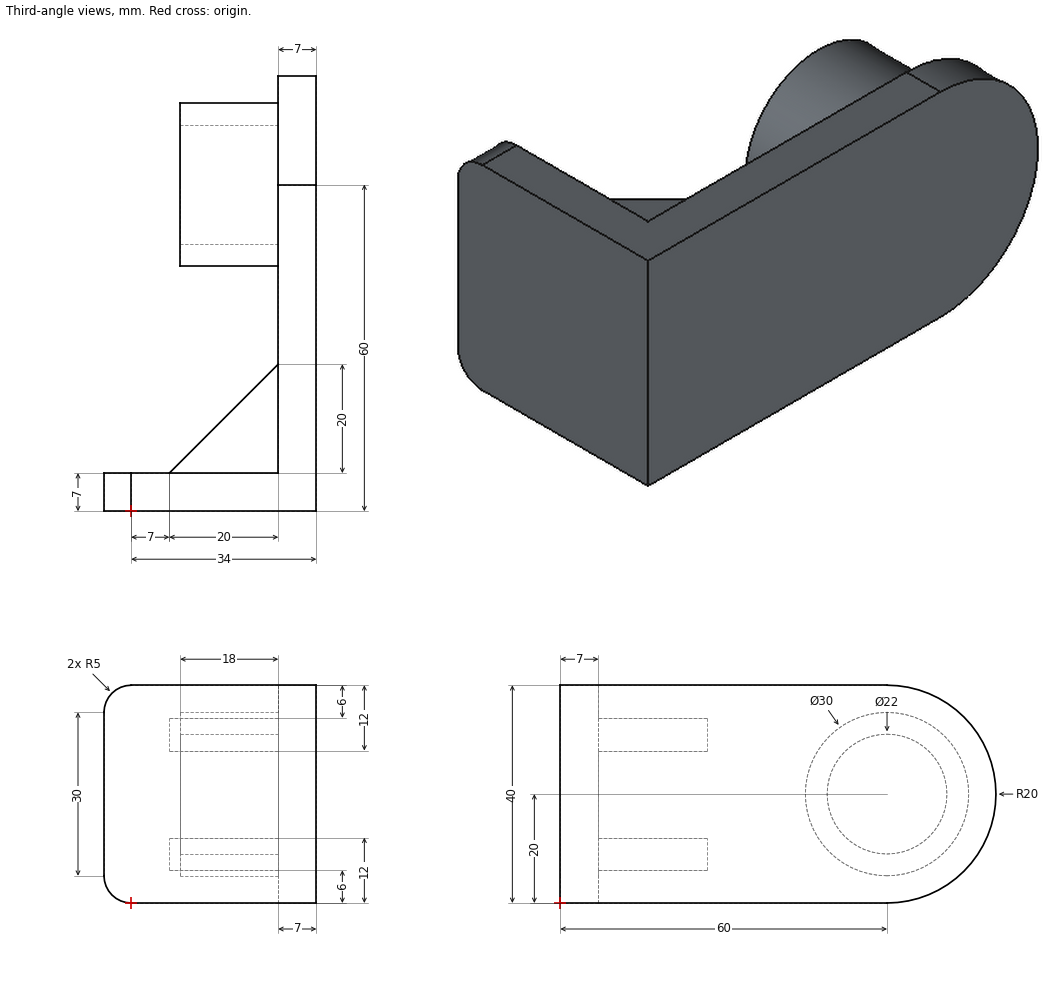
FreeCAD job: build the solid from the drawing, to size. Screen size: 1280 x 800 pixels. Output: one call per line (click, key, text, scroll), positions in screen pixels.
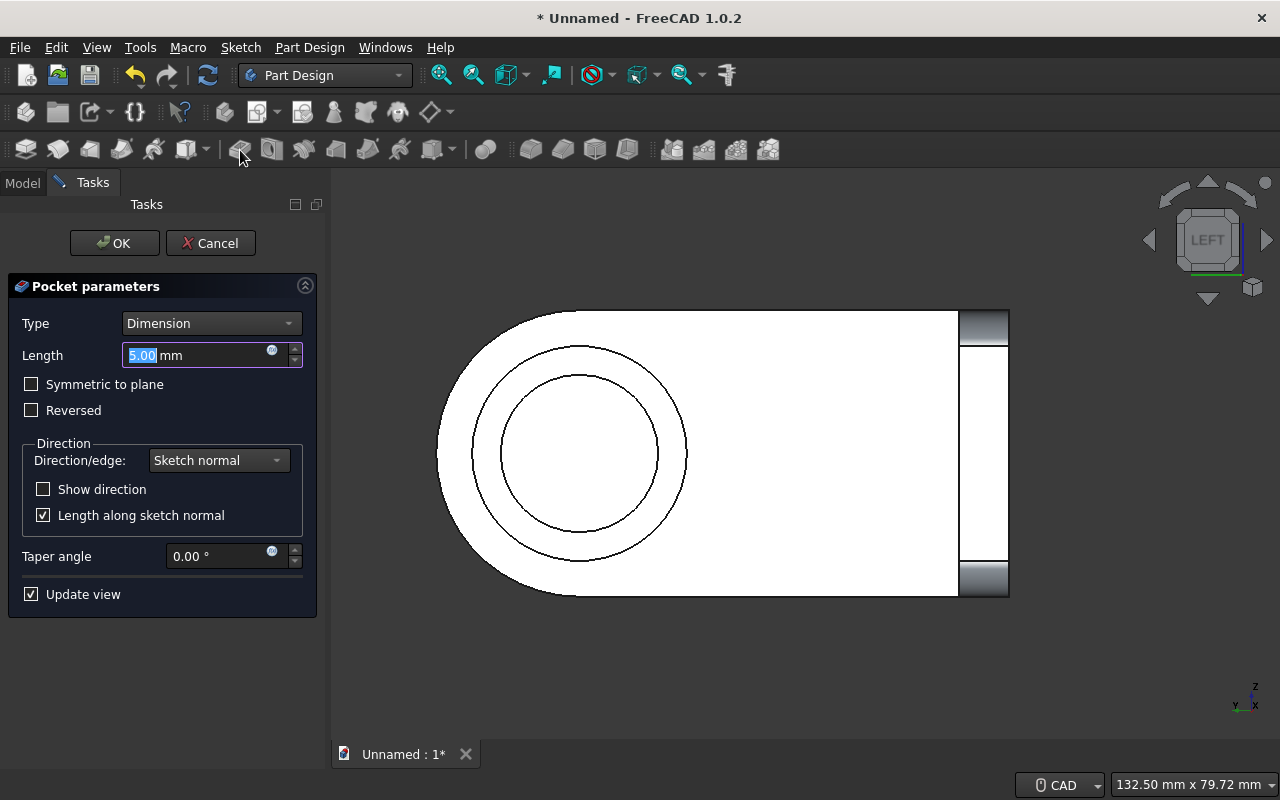
text(18)
key(Tab)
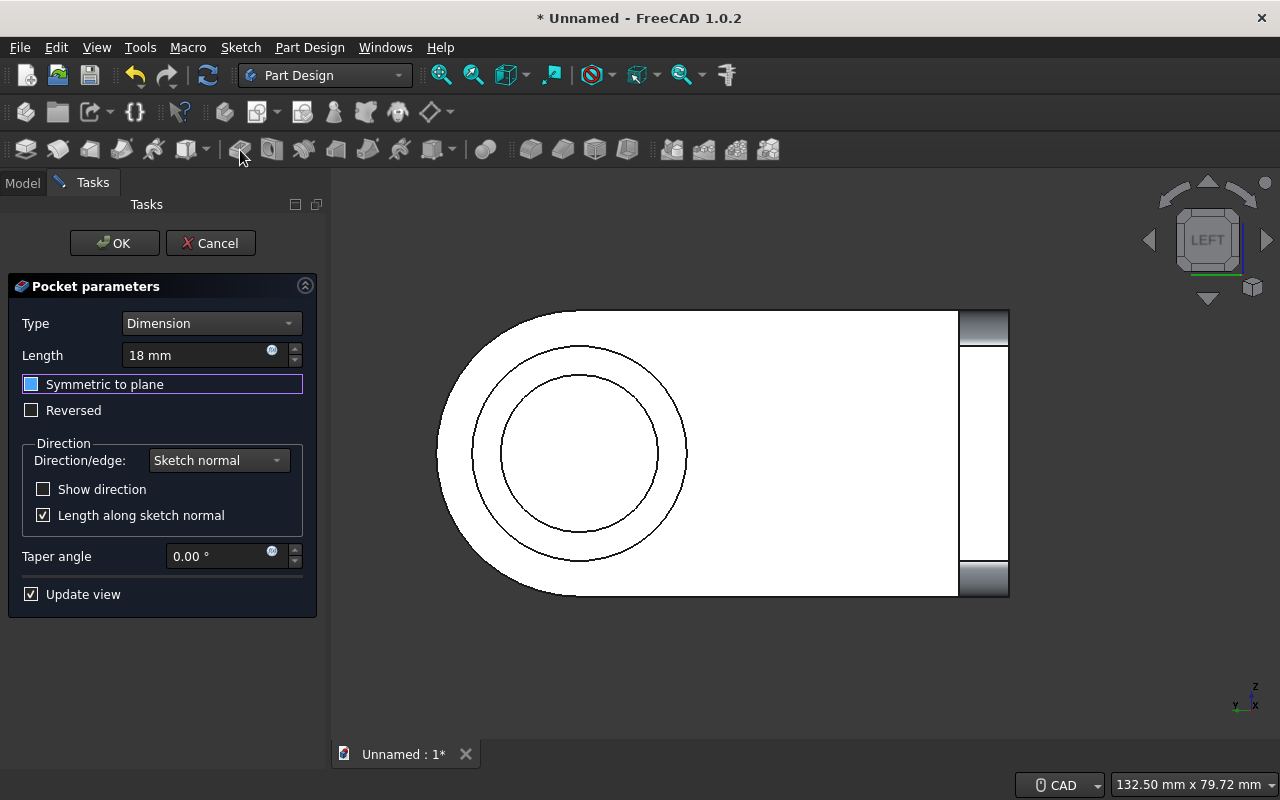
click(115, 243)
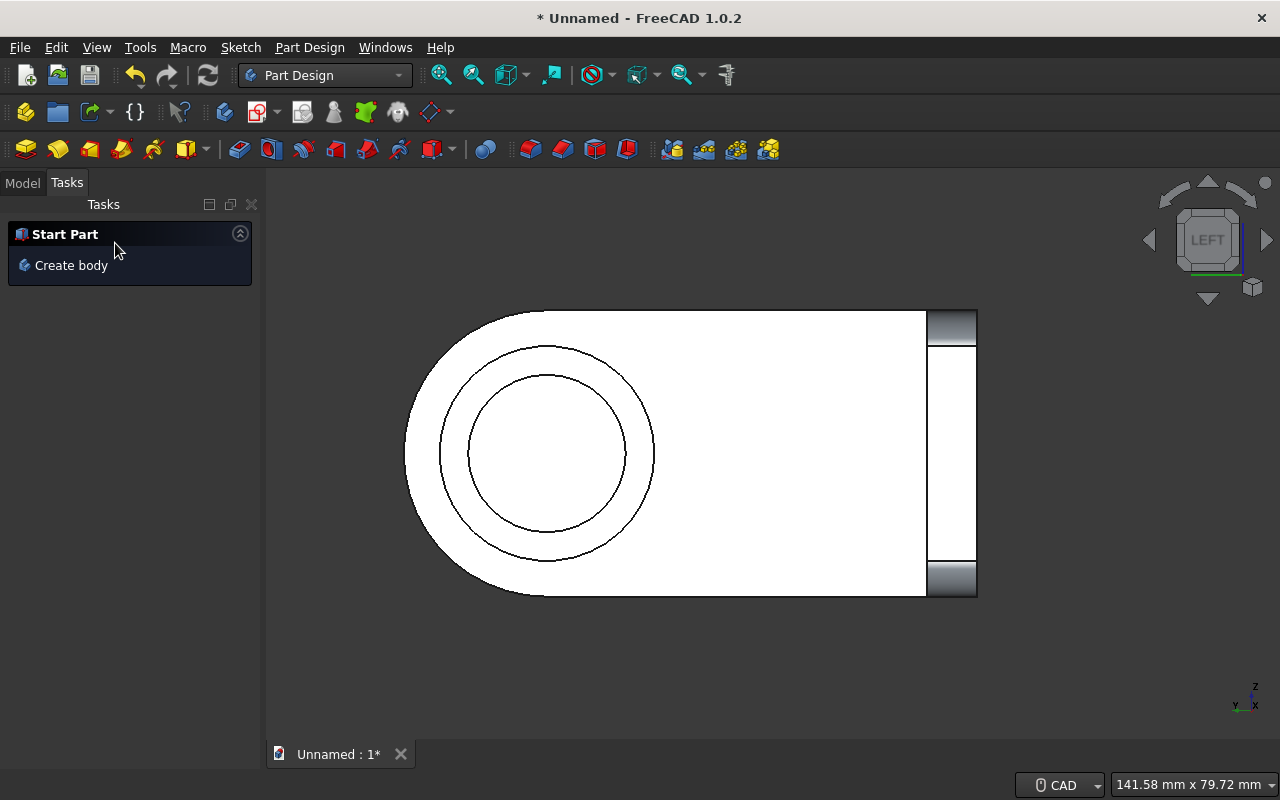
key(0)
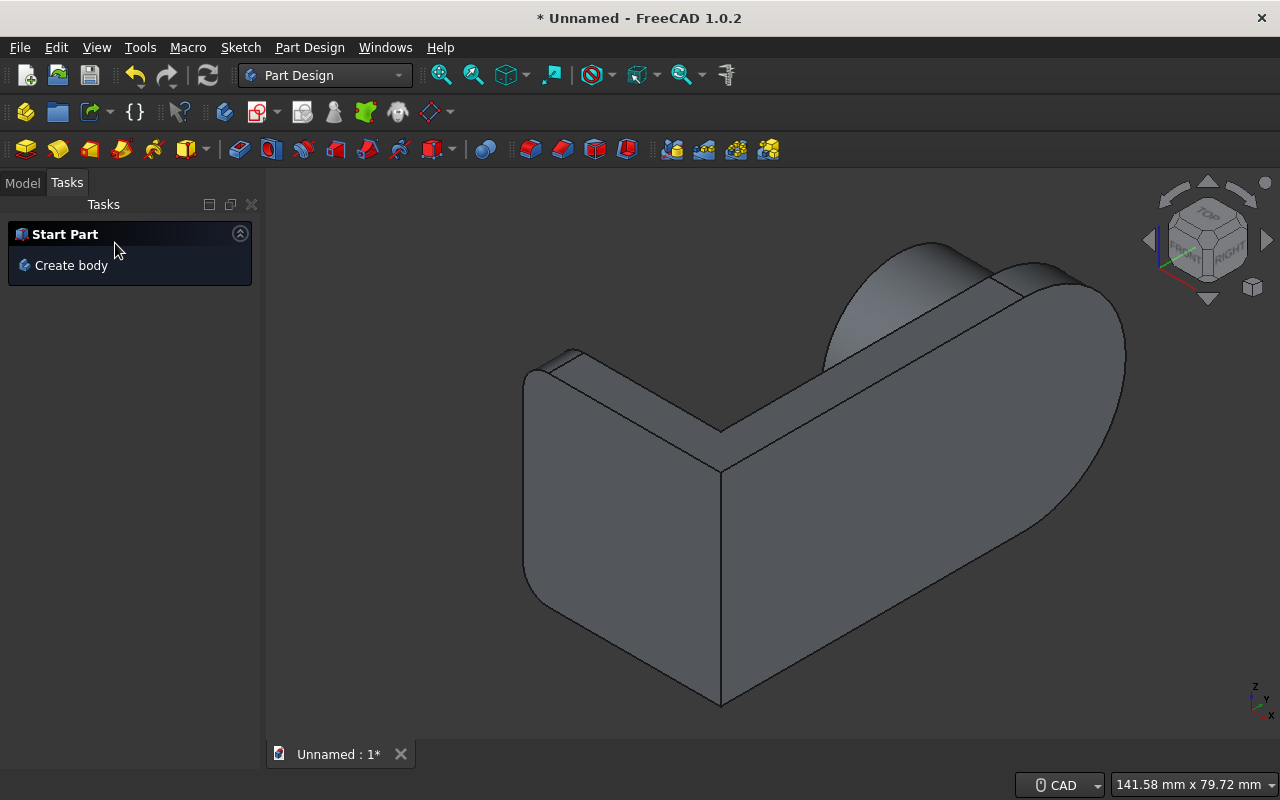
click(442, 76)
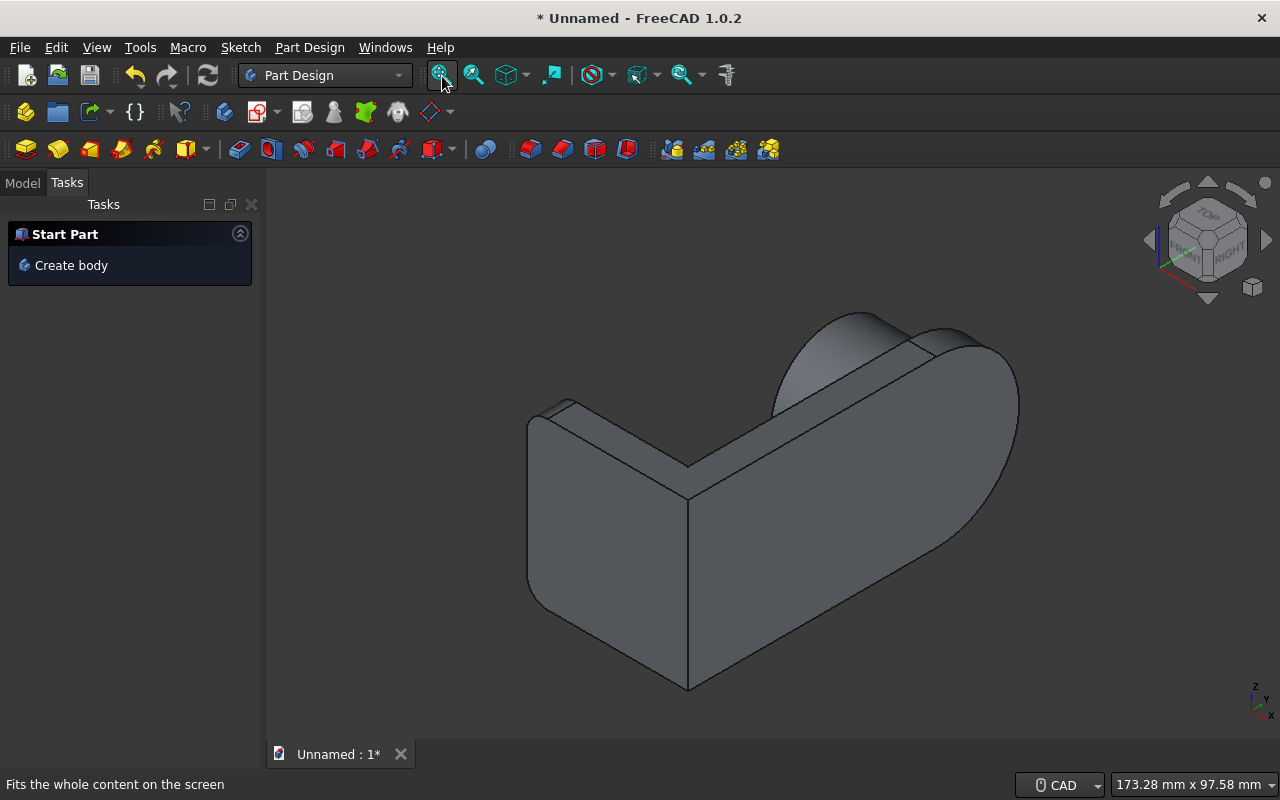
click(676, 471)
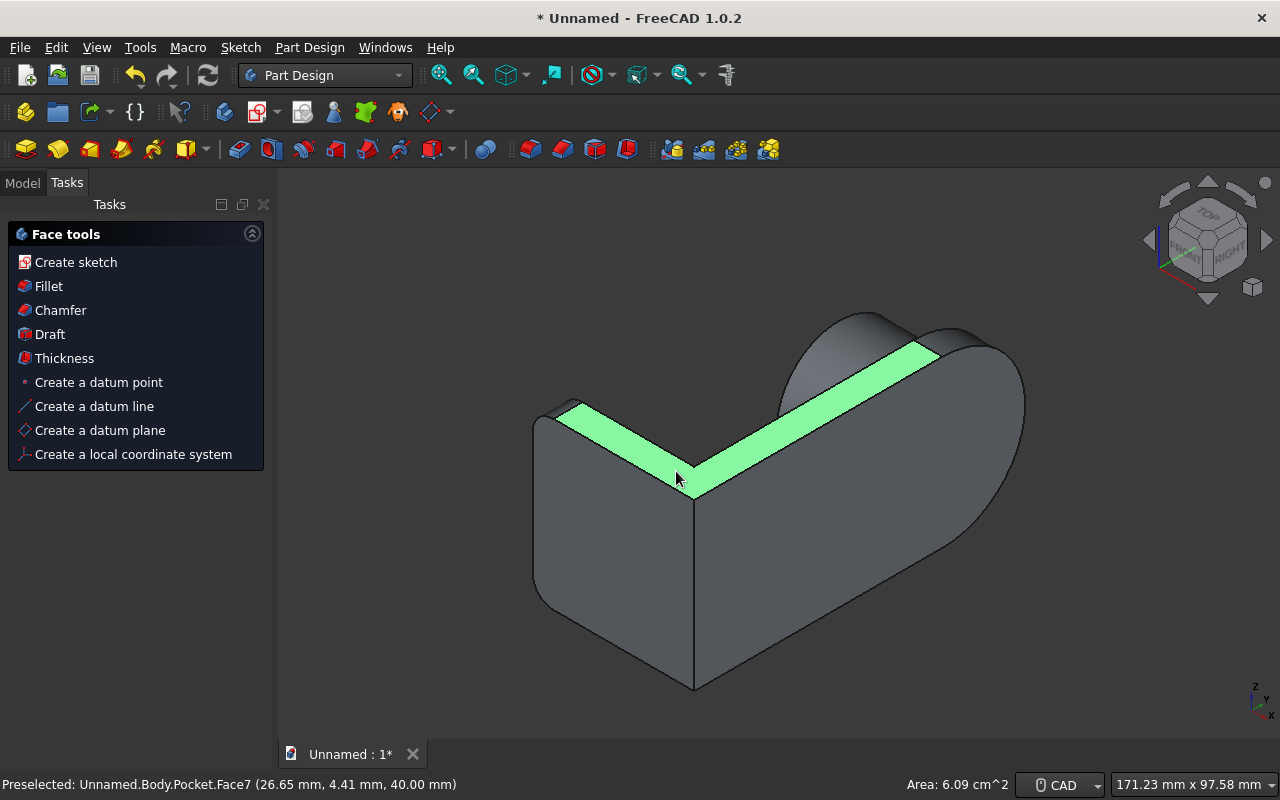
click(258, 112)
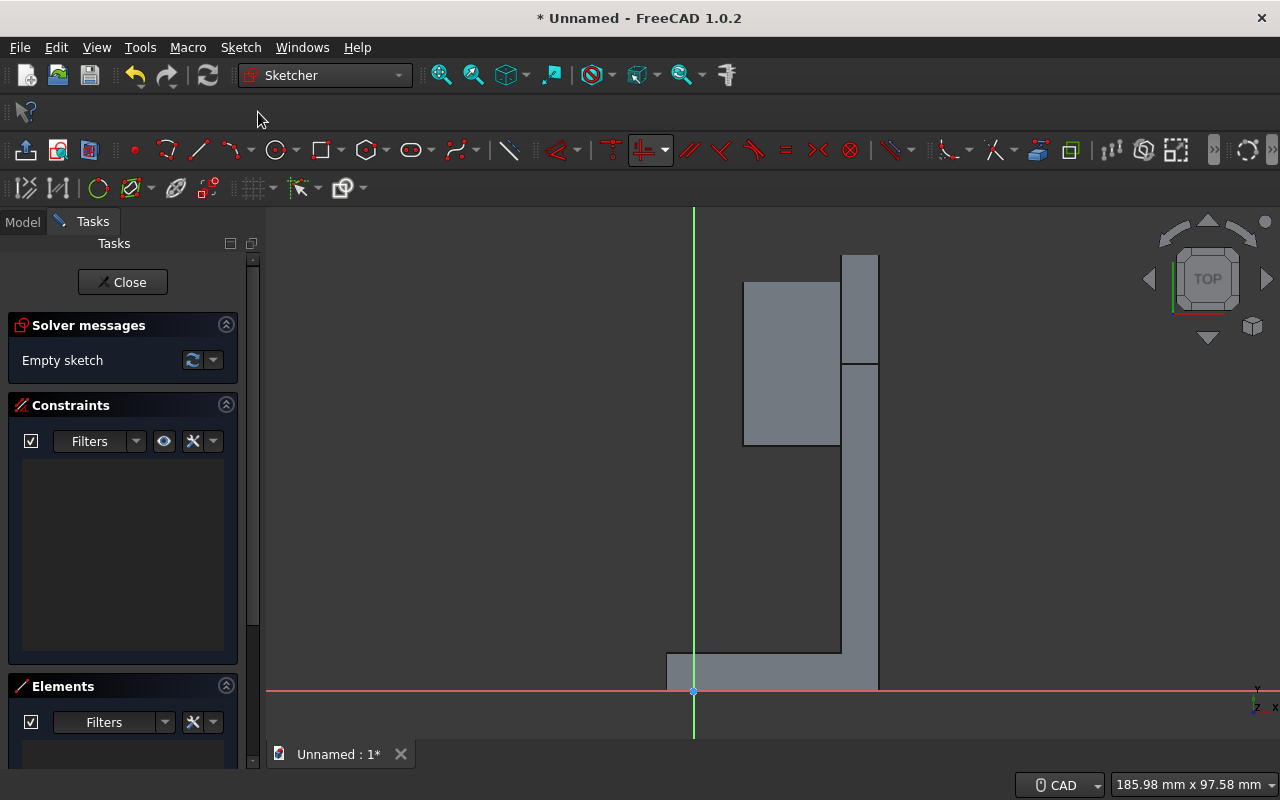
scroll(819, 711, up, 4)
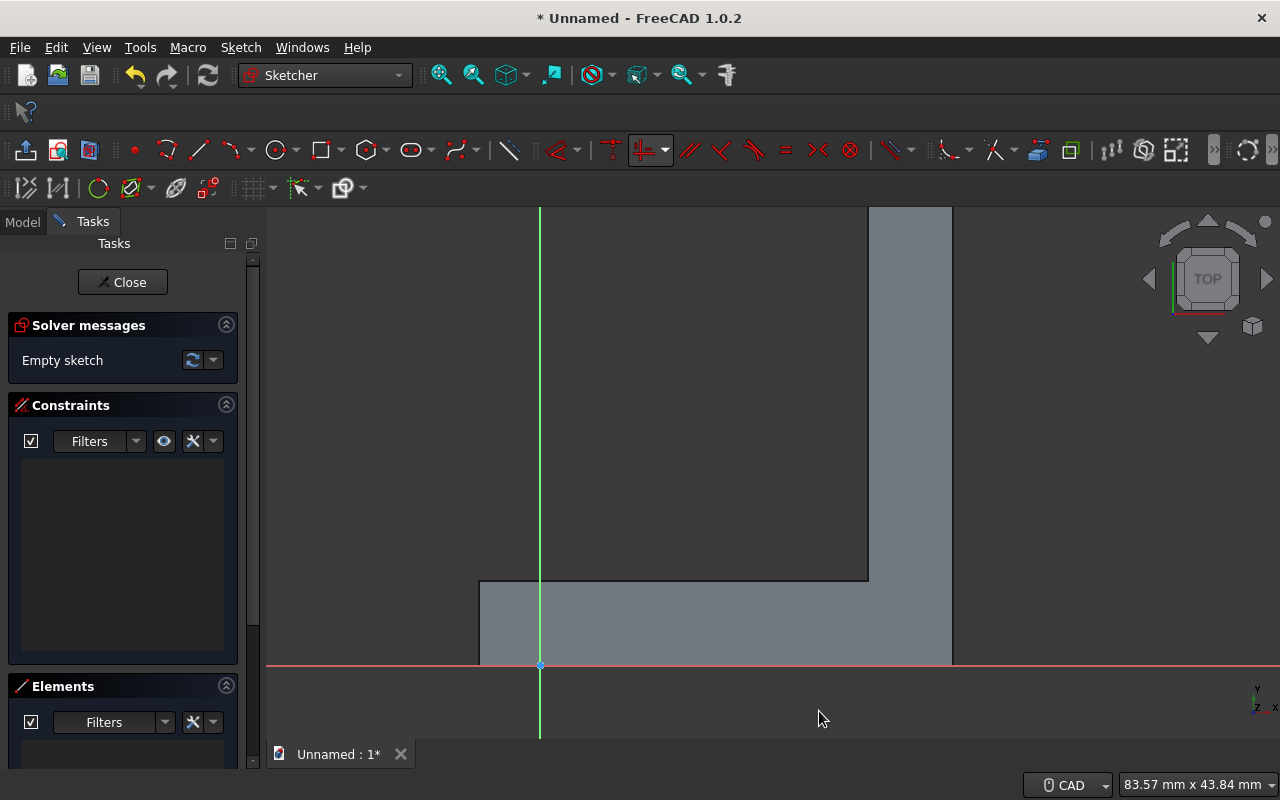
click(168, 150)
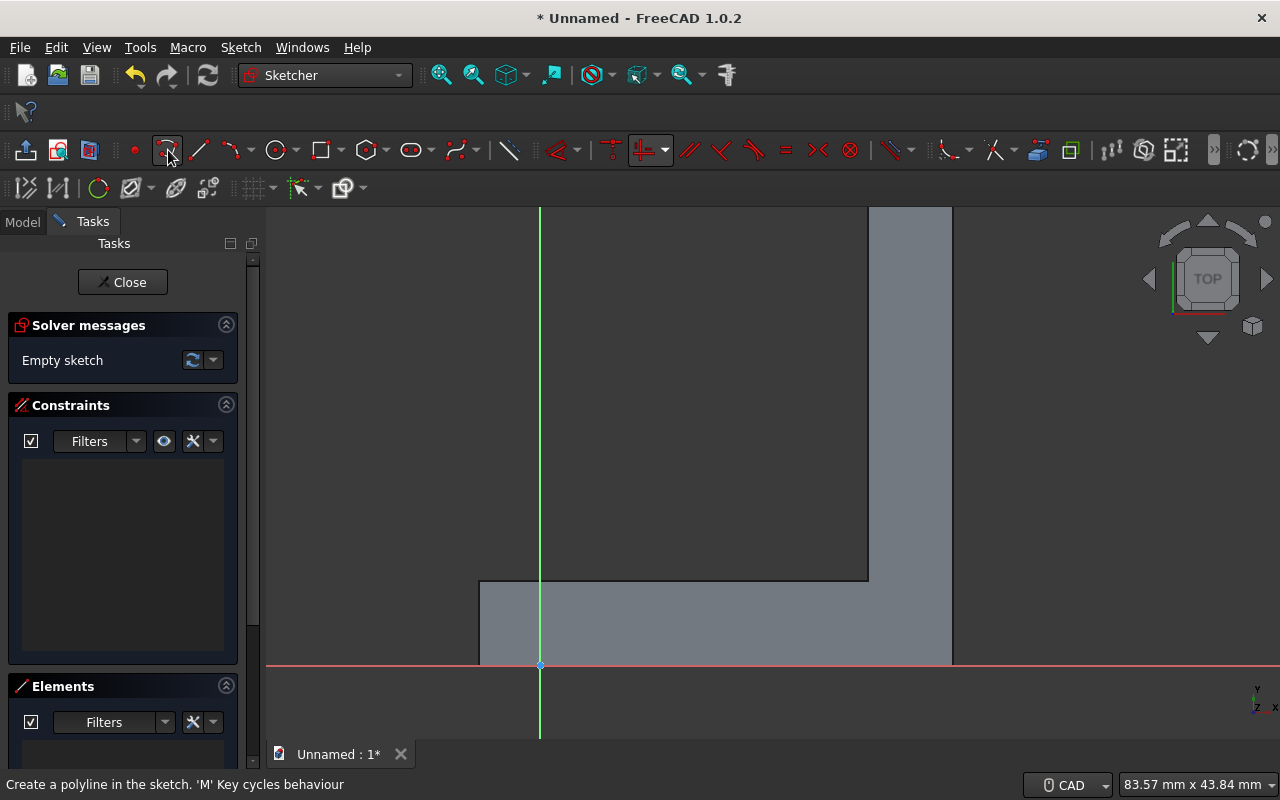
click(625, 581)
click(868, 581)
click(868, 338)
click(625, 582)
key(Escape)
key(Escape)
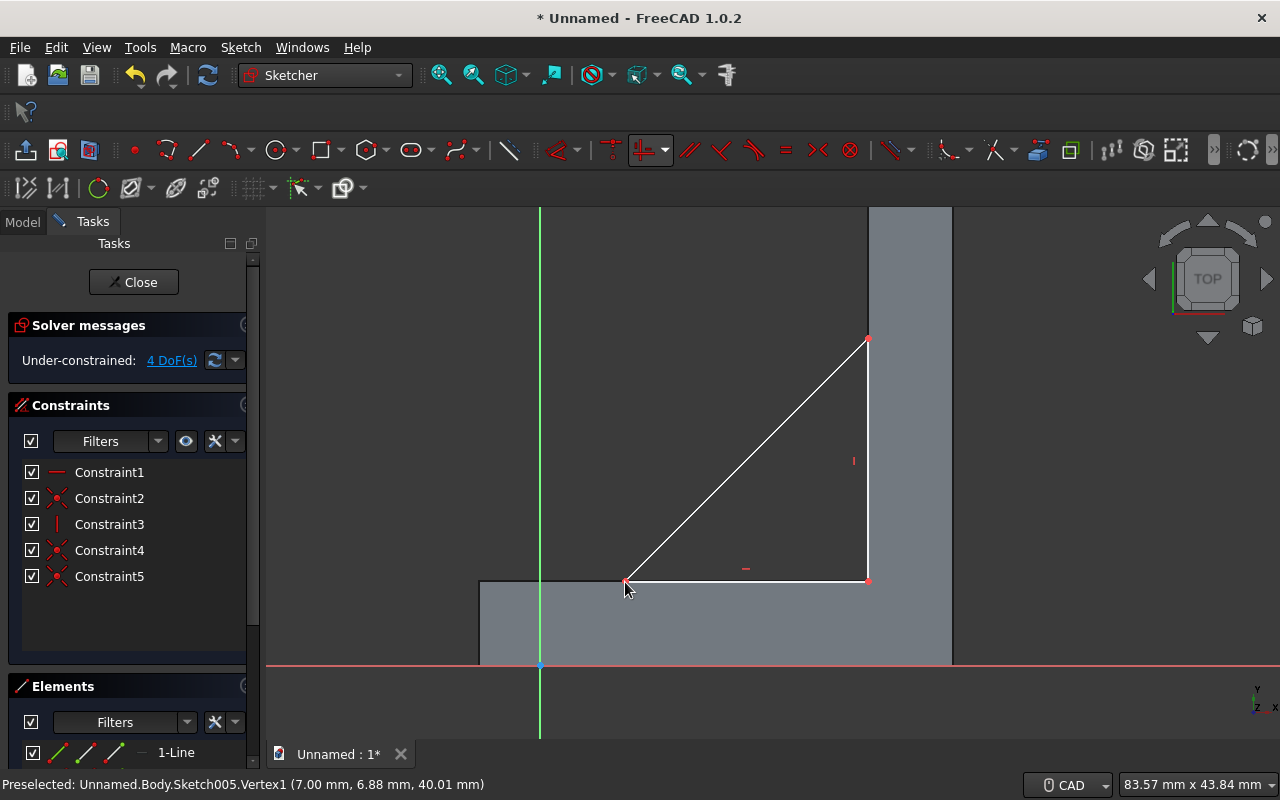
click(556, 150)